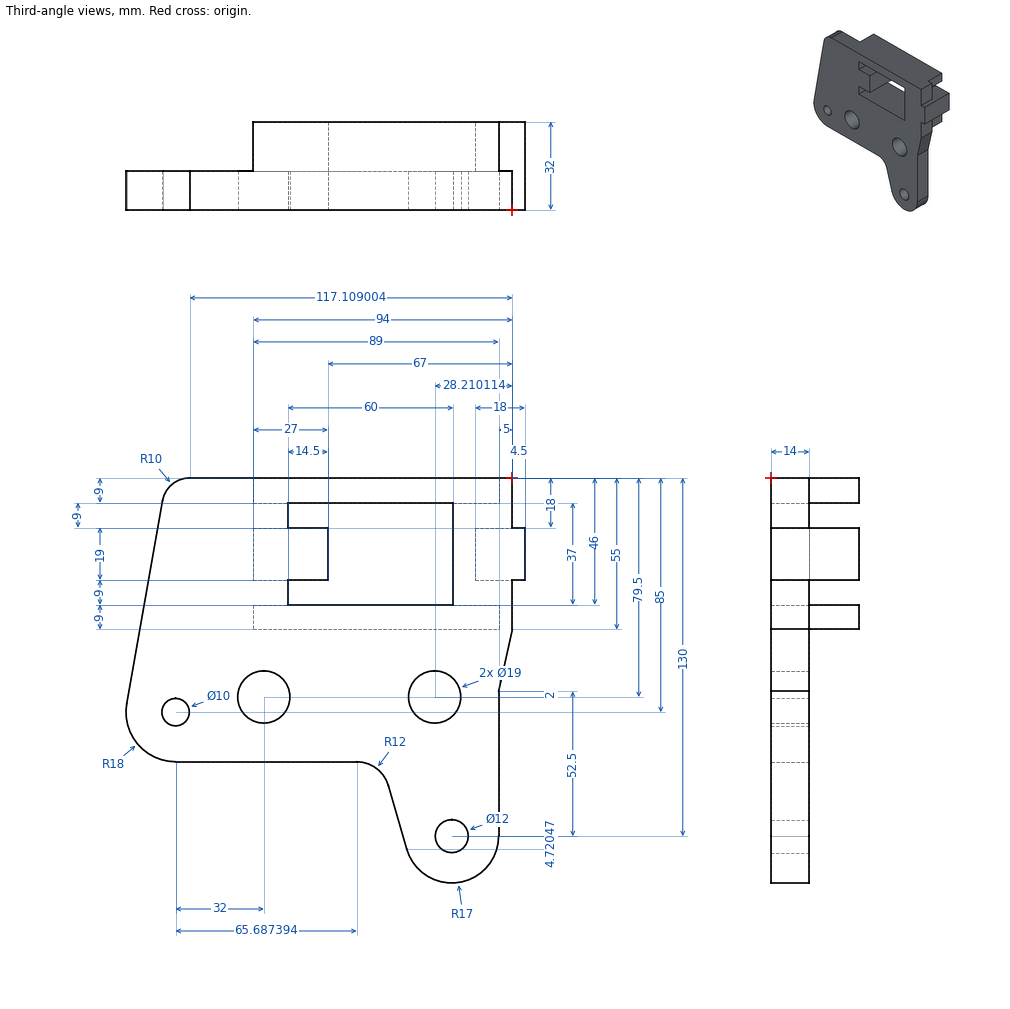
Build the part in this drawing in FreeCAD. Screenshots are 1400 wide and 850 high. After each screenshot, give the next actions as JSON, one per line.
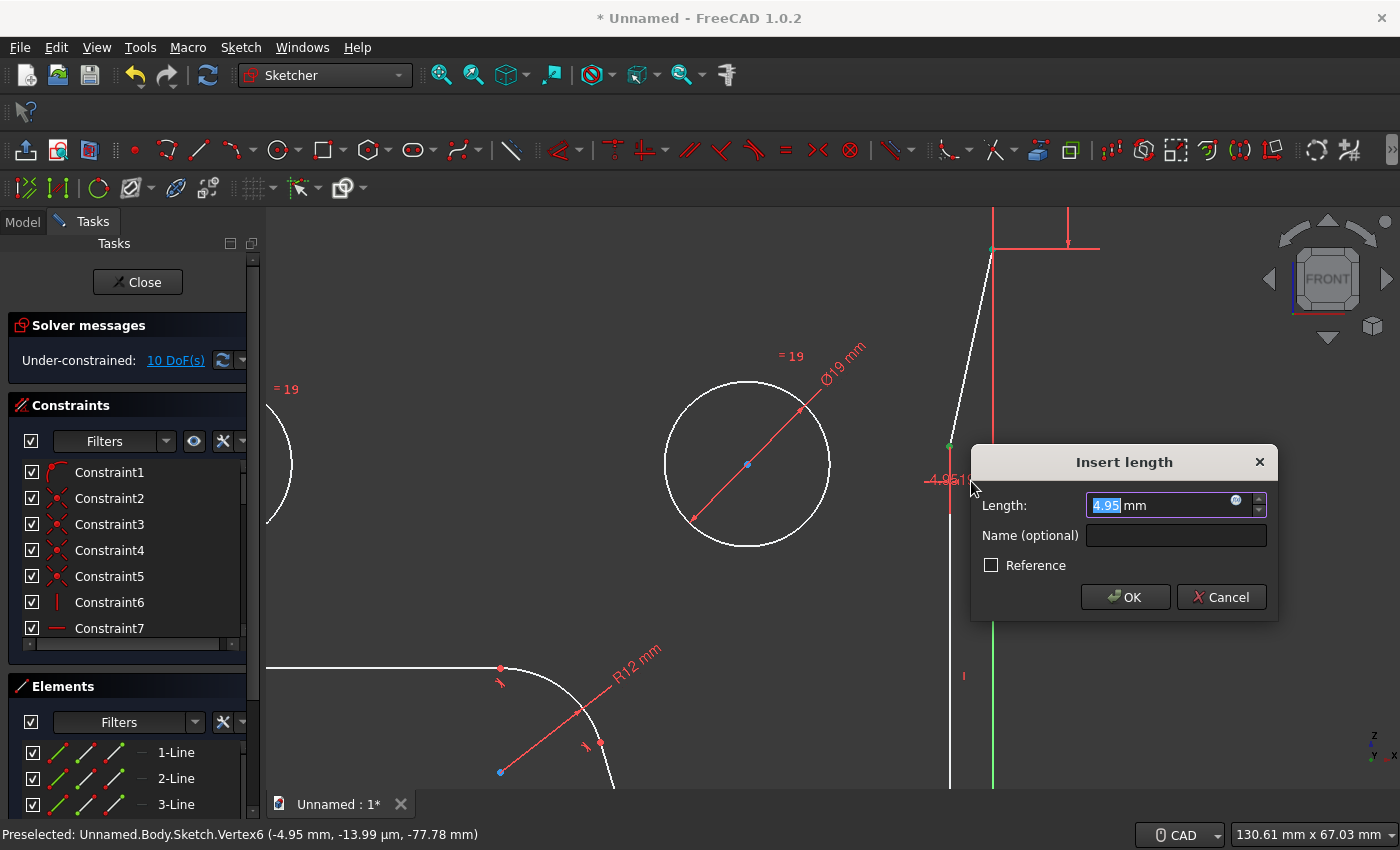
{"action": "type", "text": "5"}
{"action": "key", "text": "Return"}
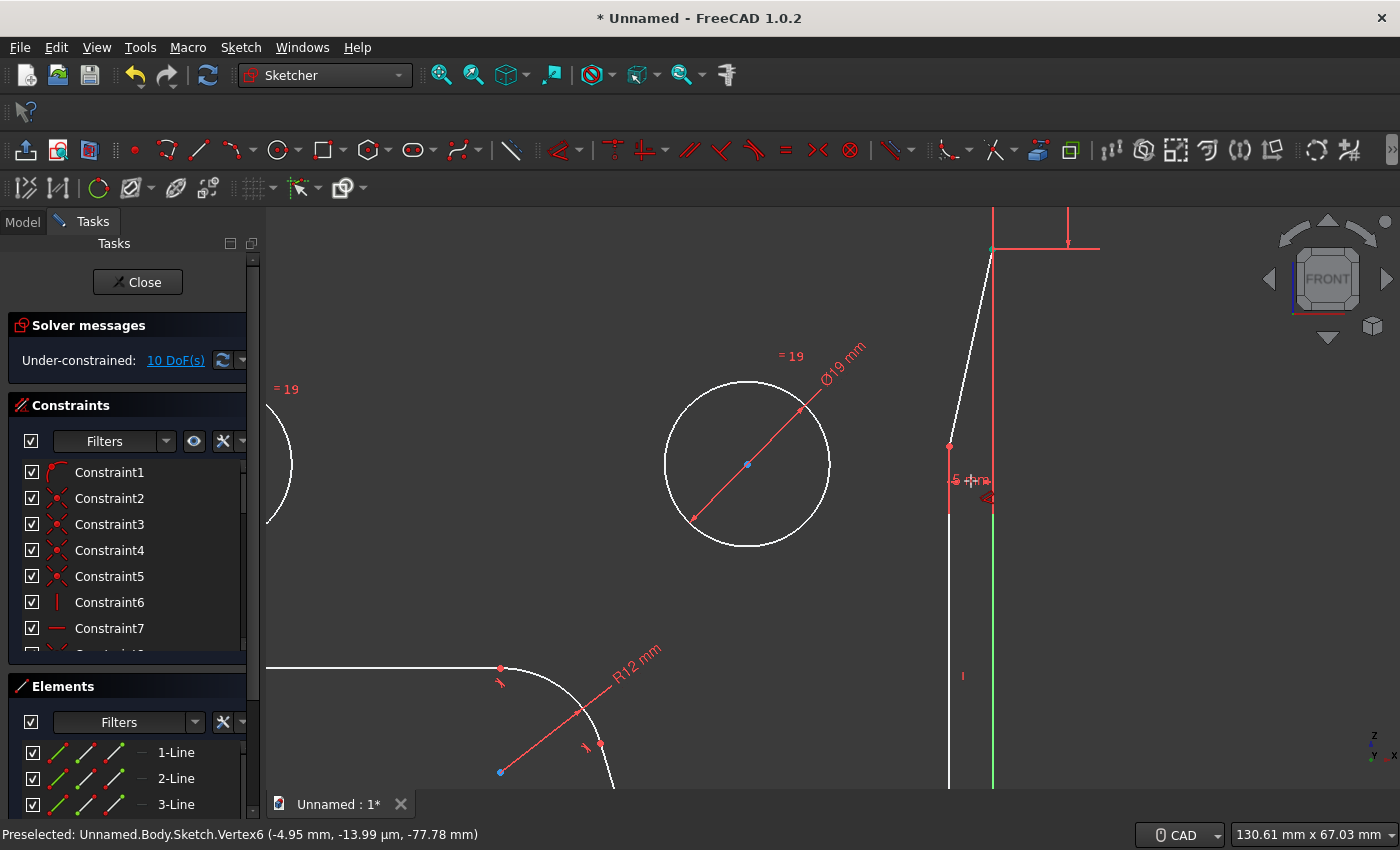
{"action": "scroll", "coordinate": [928, 536], "scroll_direction": "down", "scroll_amount": 6}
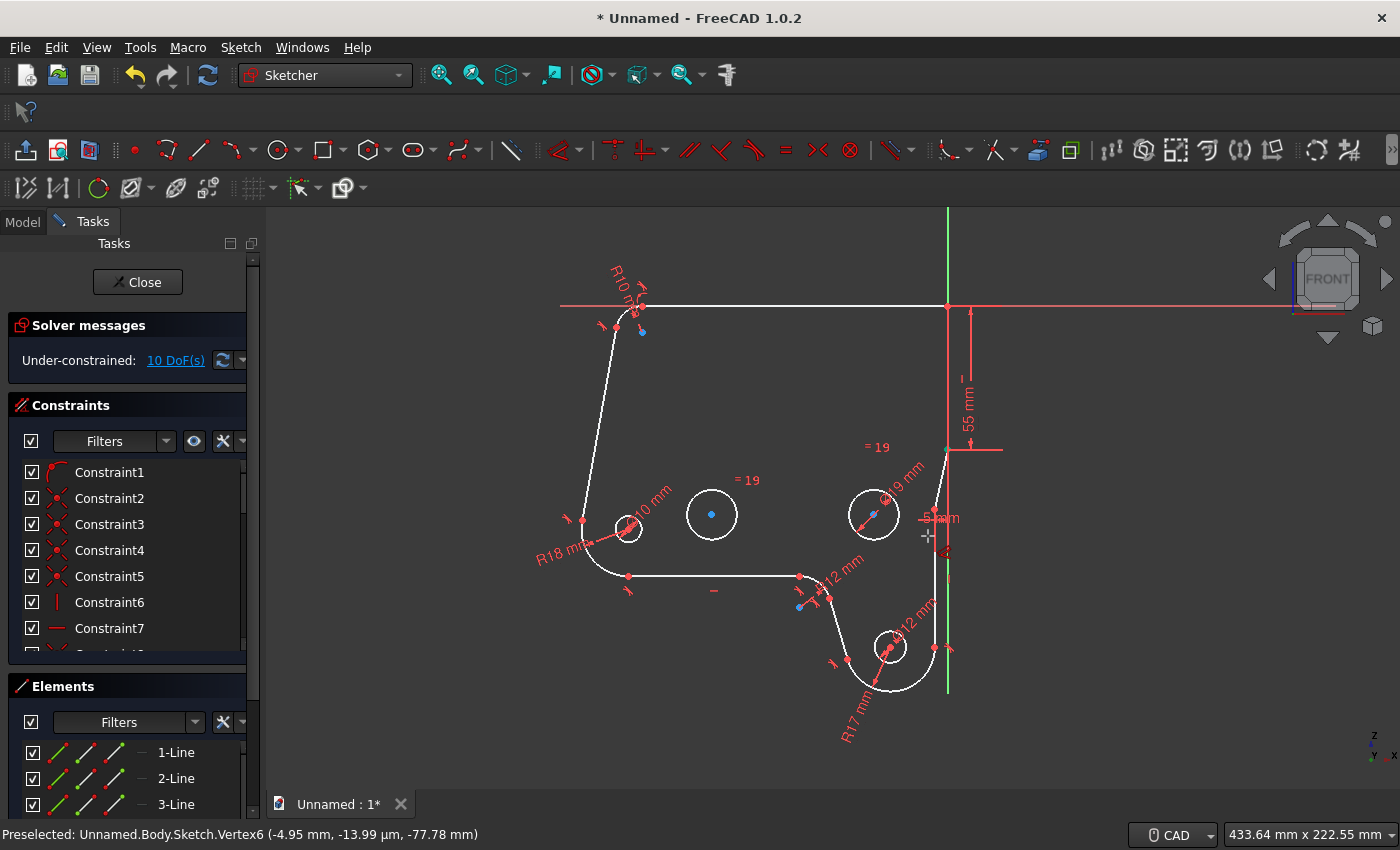
{"action": "left_click", "coordinate": [629, 529]}
{"action": "left_click", "coordinate": [982, 366]}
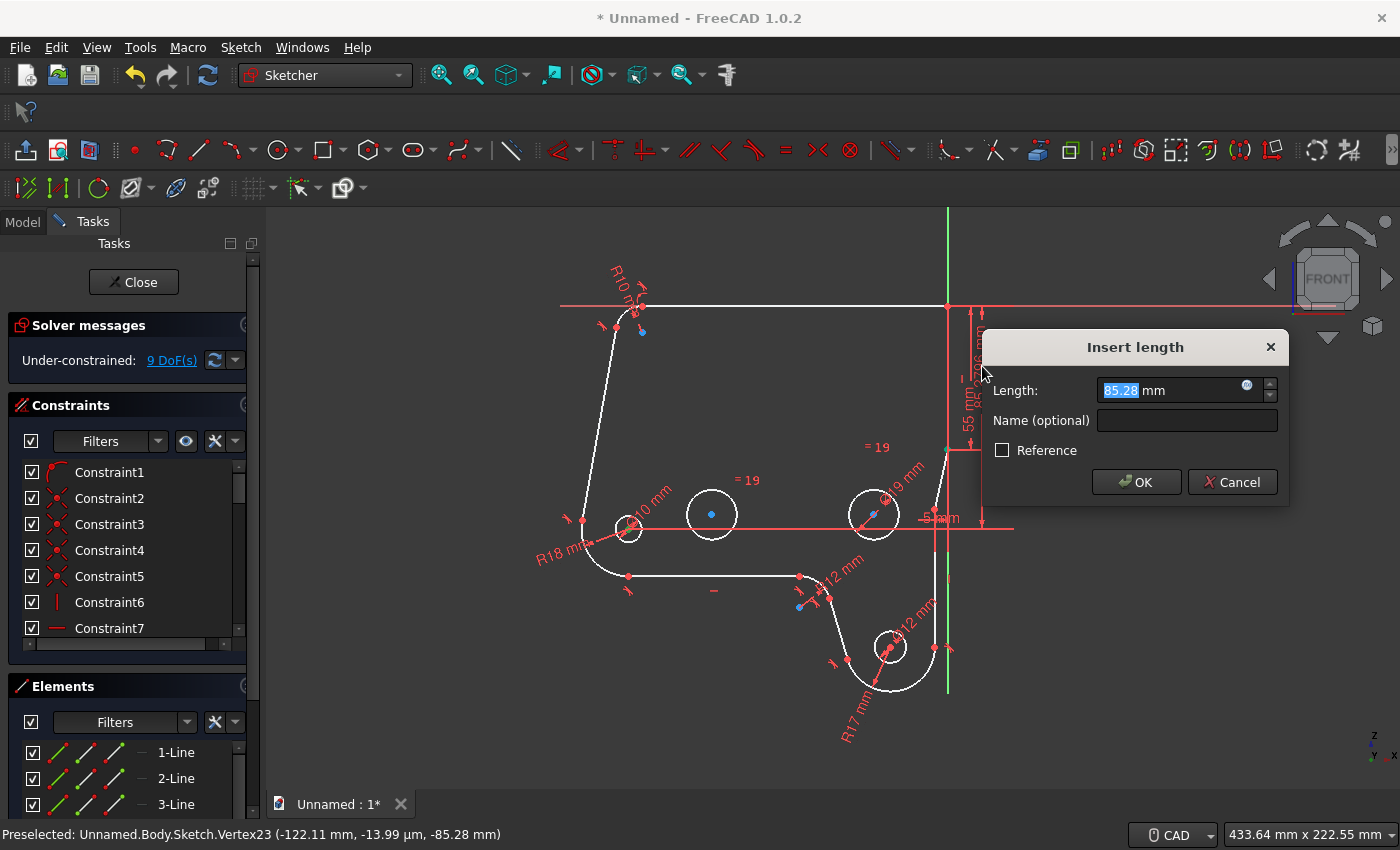
{"action": "type", "text": "85"}
{"action": "key", "text": "Return"}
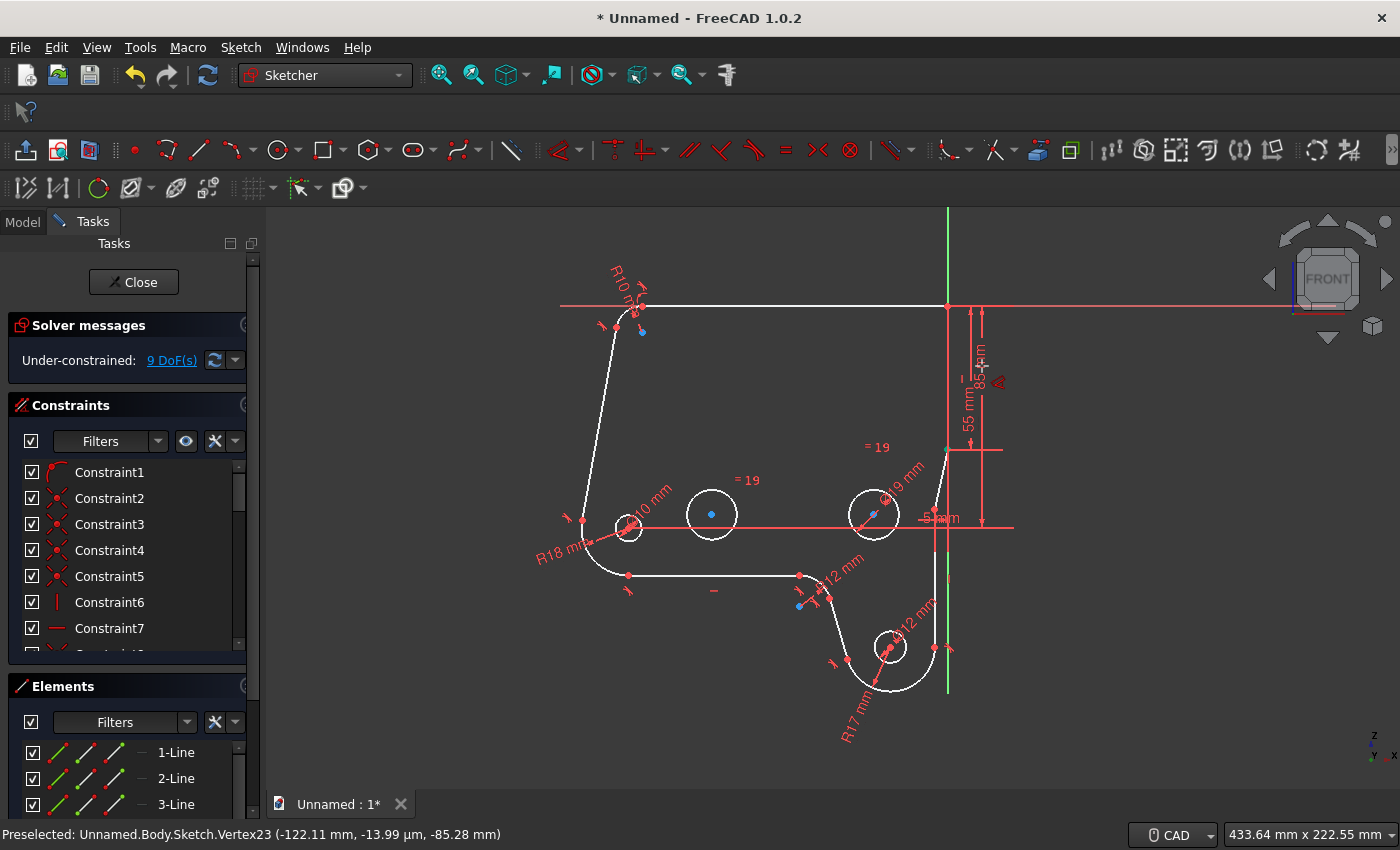
{"action": "scroll", "coordinate": [935, 510], "scroll_direction": "up", "scroll_amount": 11}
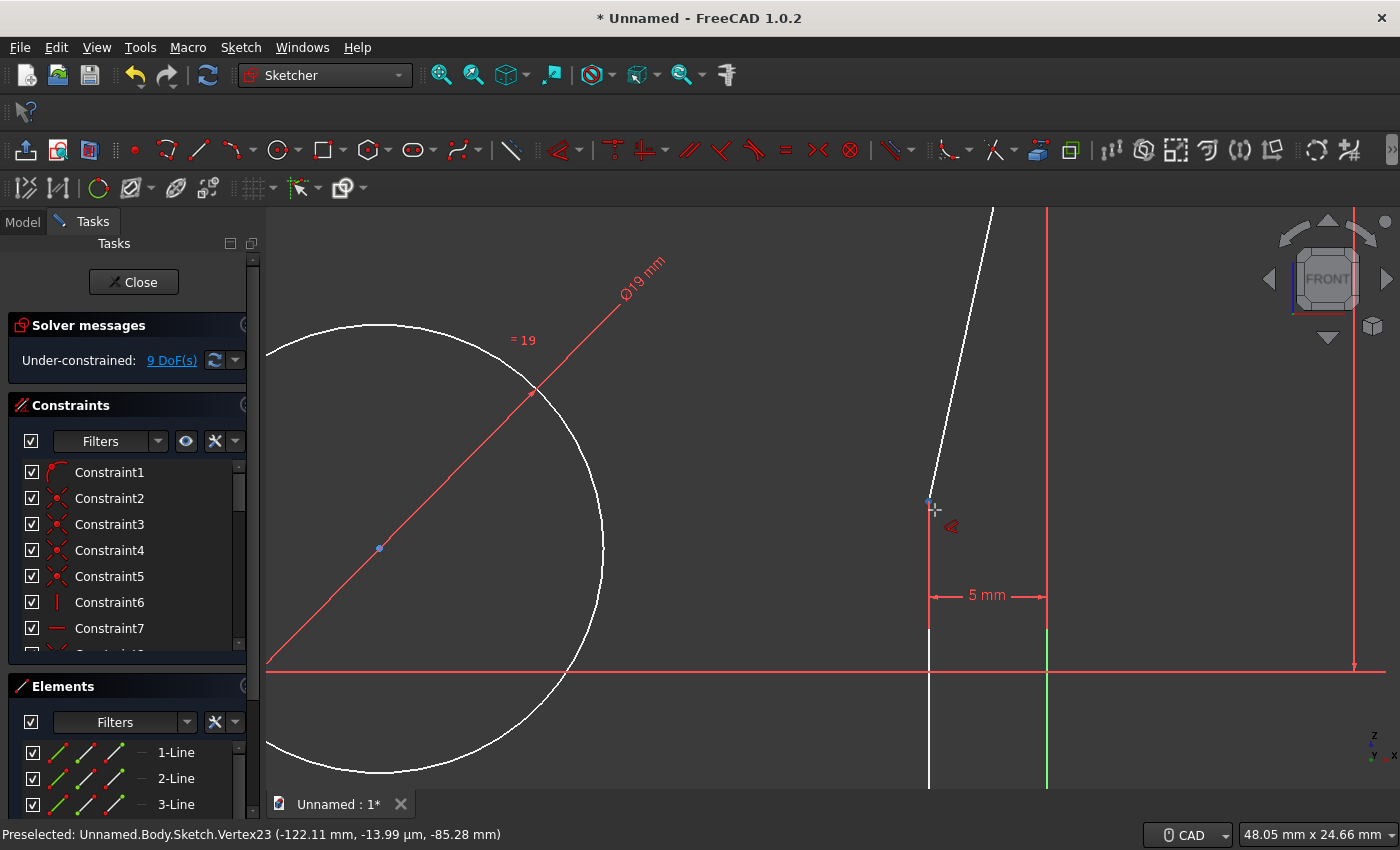
{"action": "left_click", "coordinate": [929, 502]}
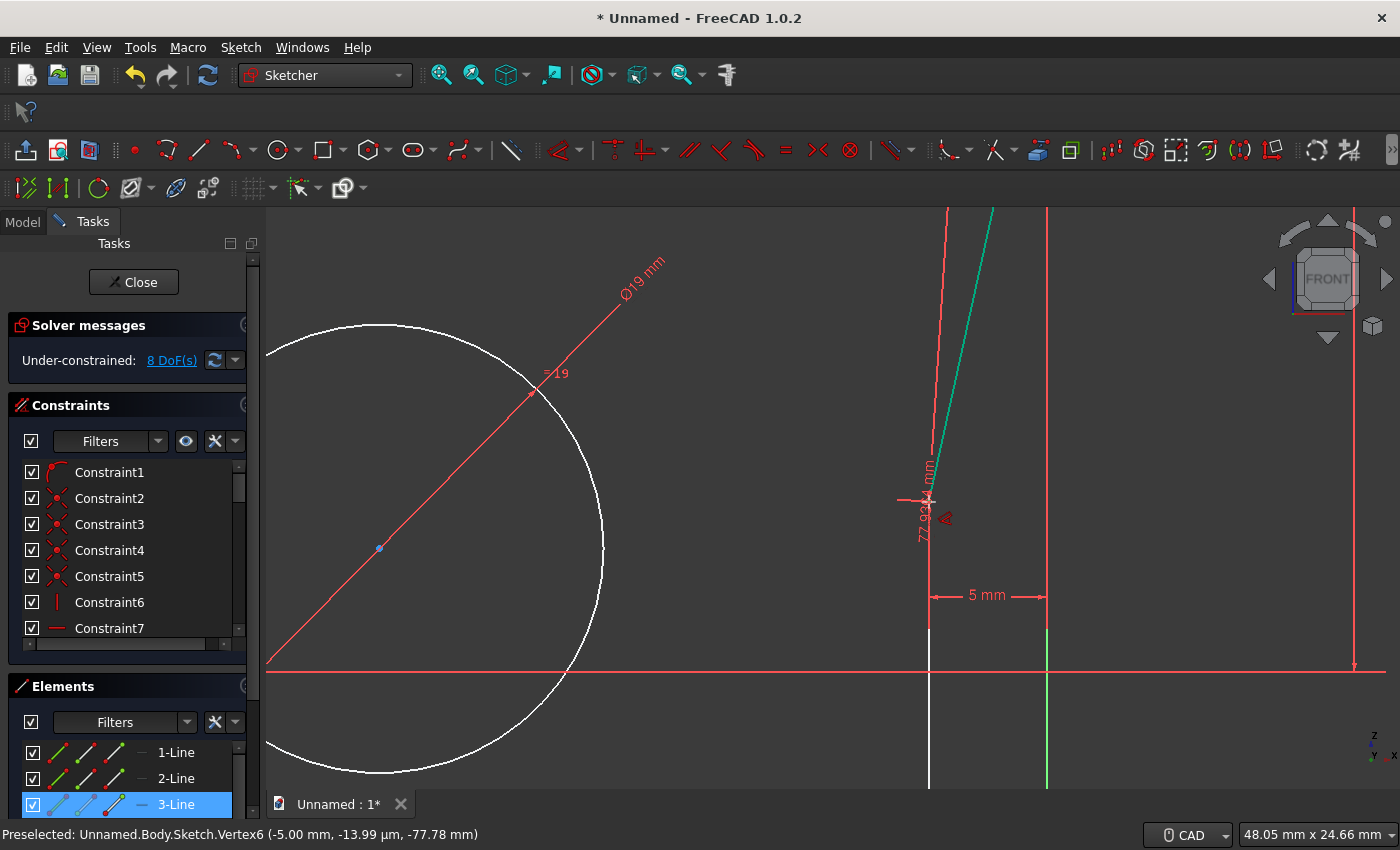
{"action": "left_click", "coordinate": [379, 549]}
{"action": "left_click", "coordinate": [963, 525]}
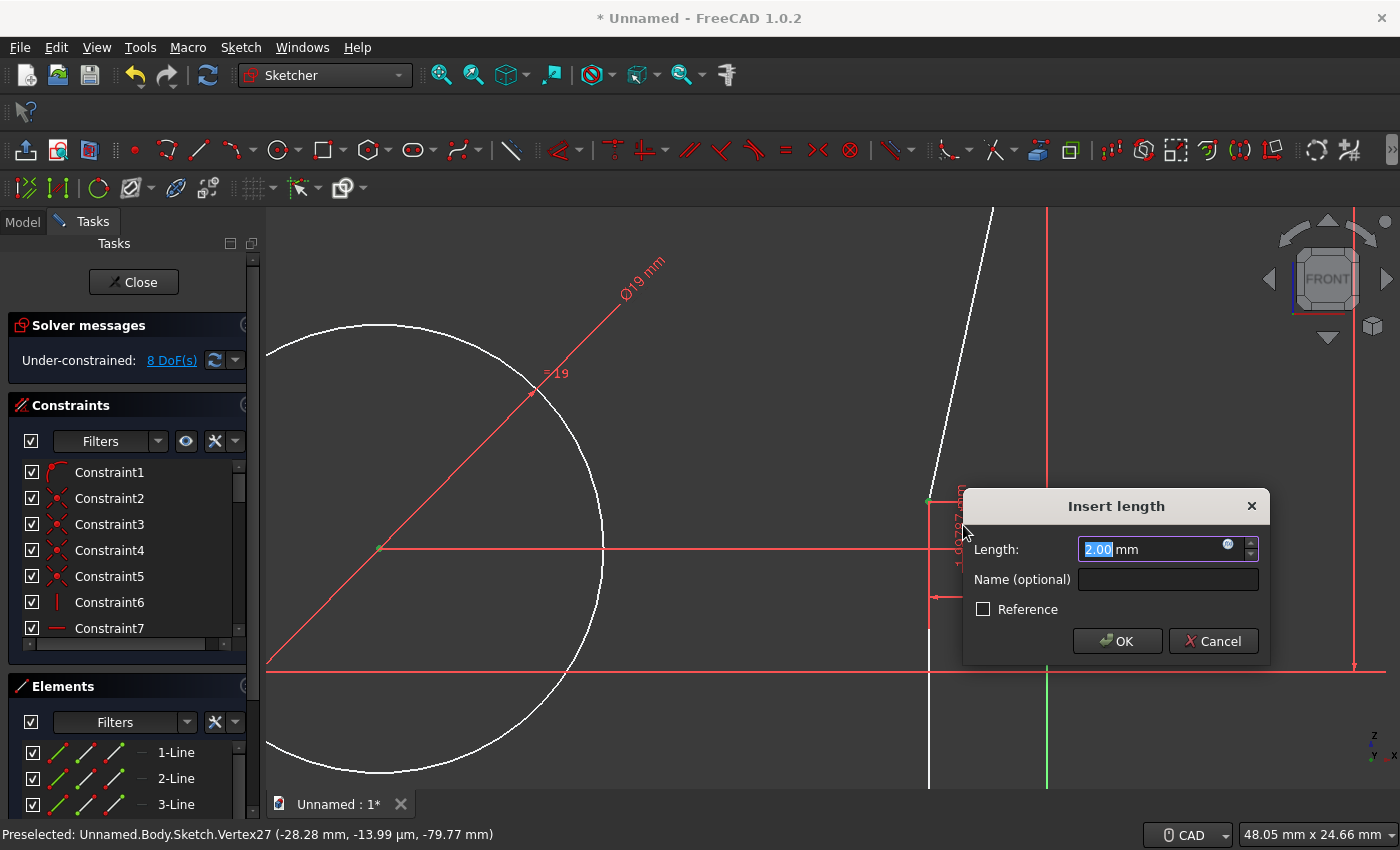
{"action": "type", "text": "2"}
{"action": "key", "text": "Return"}